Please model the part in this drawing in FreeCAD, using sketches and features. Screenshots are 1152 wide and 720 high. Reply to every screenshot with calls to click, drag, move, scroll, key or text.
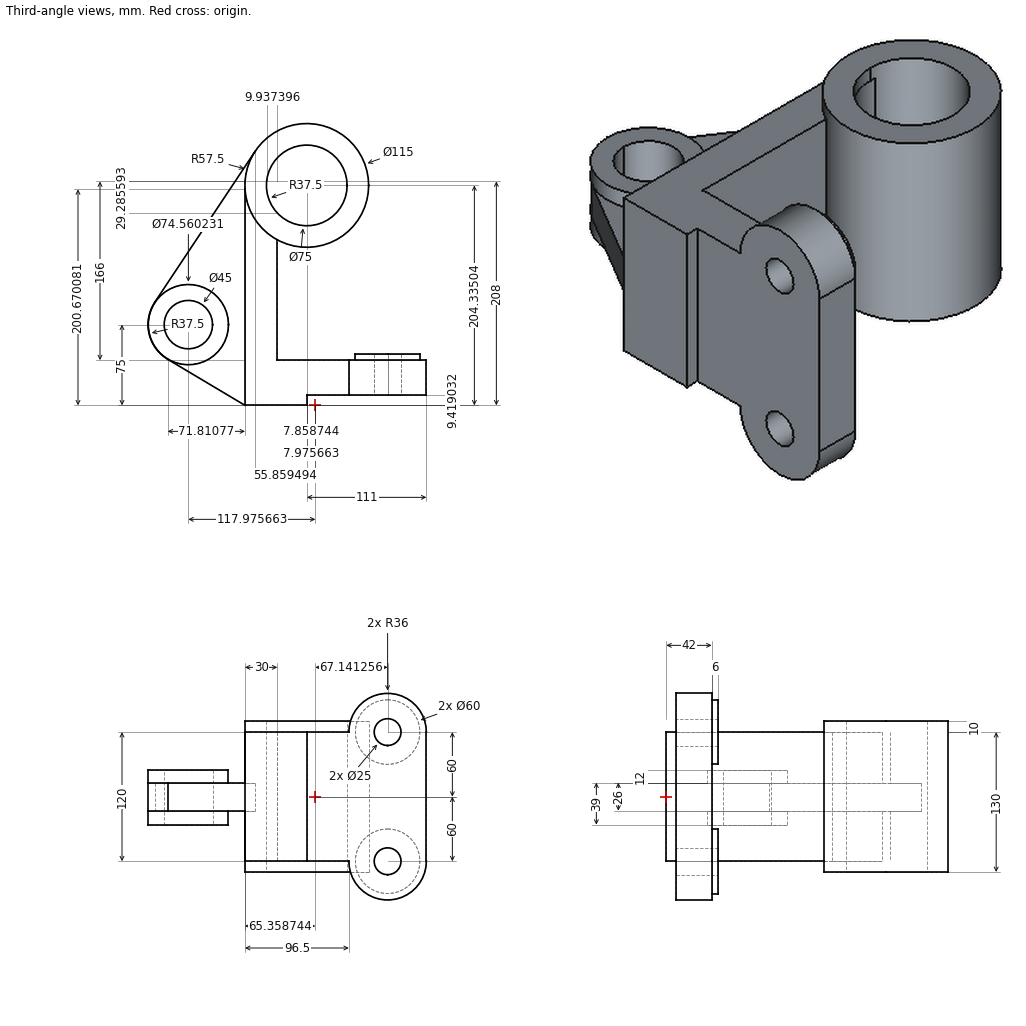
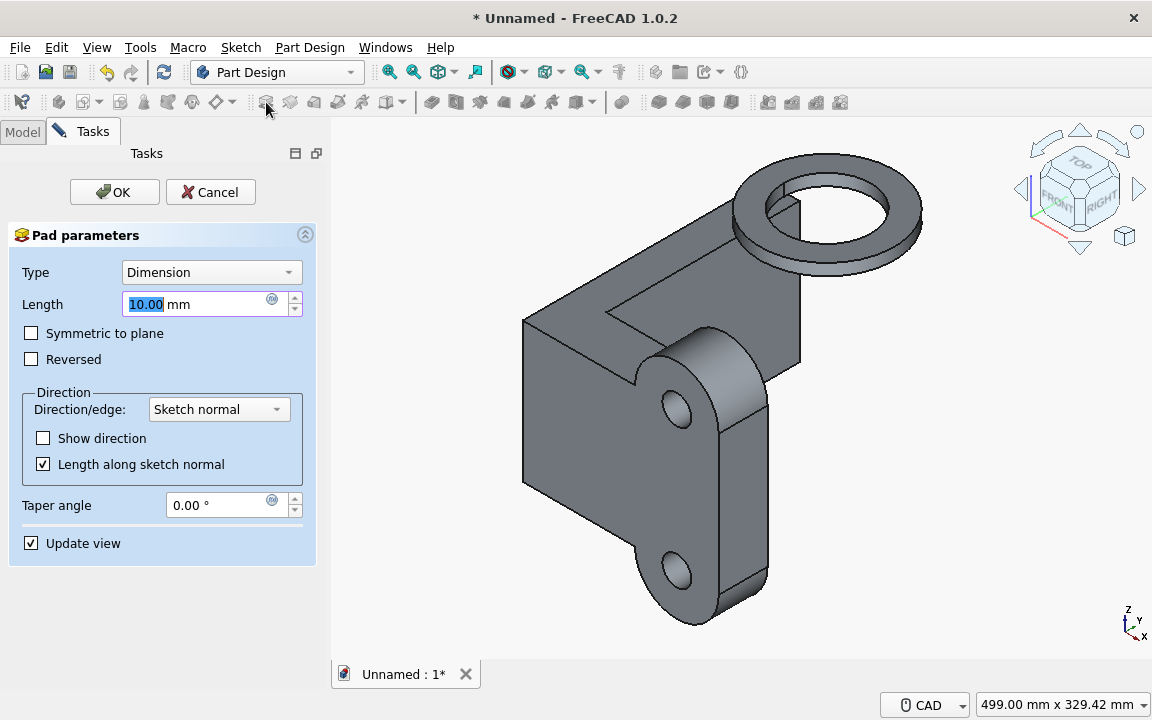
click(212, 272)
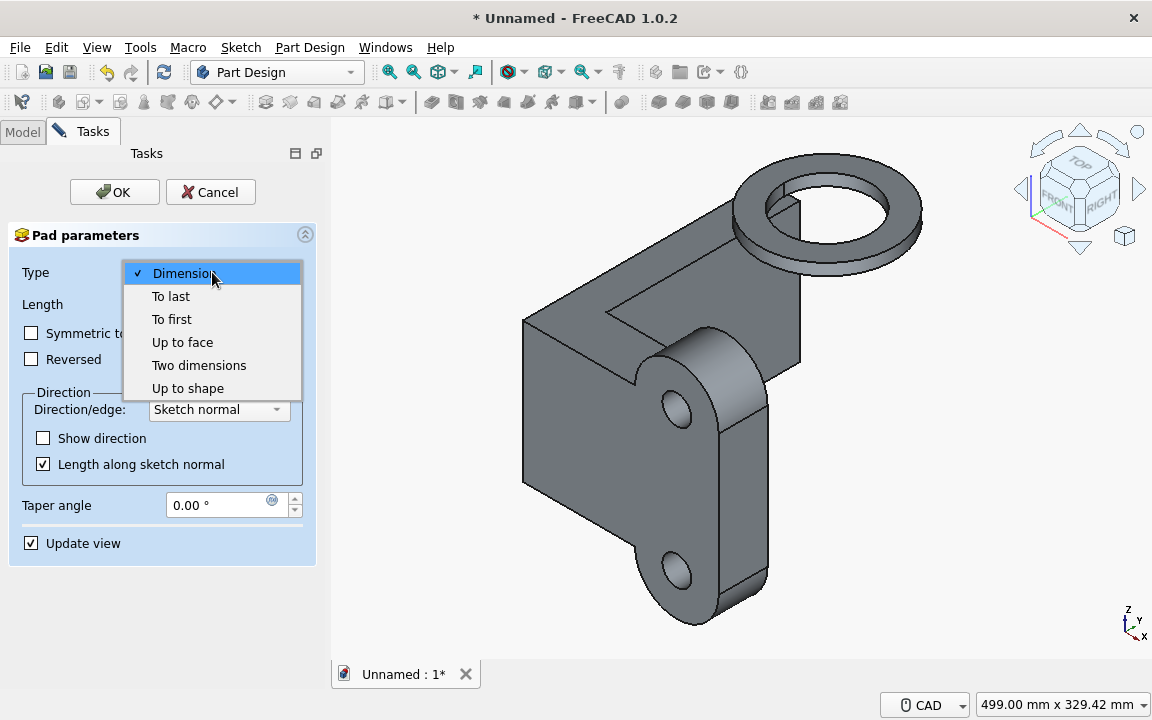
click(212, 366)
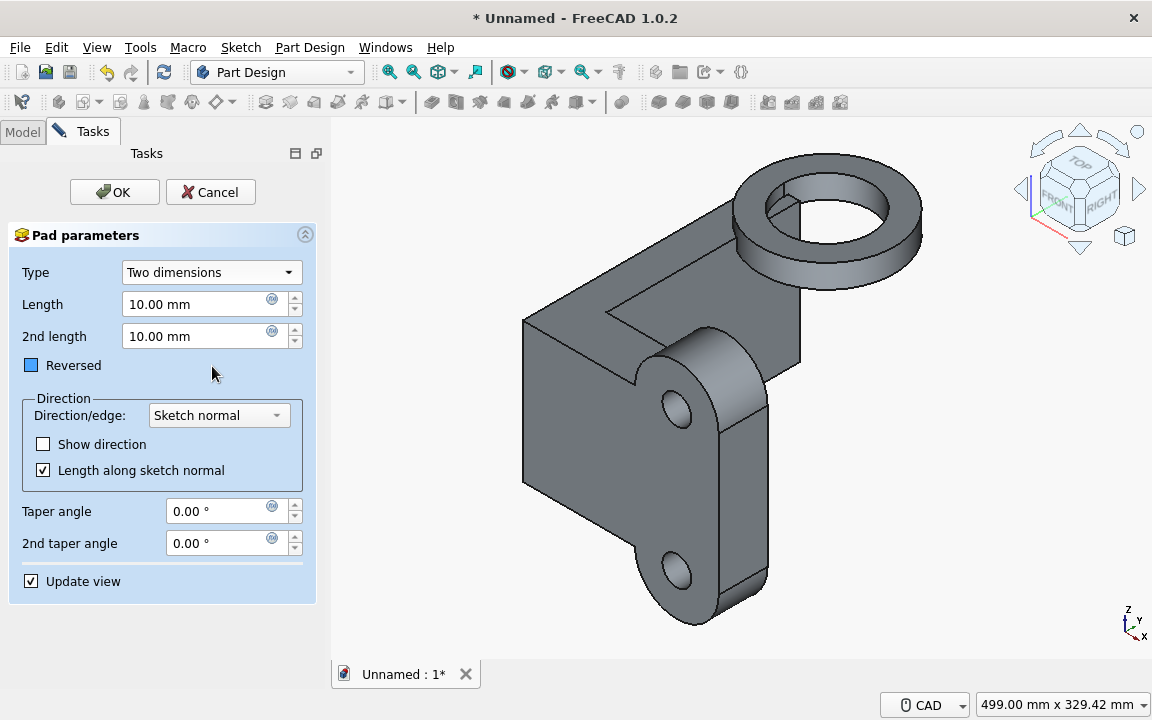
triple_click(204, 304)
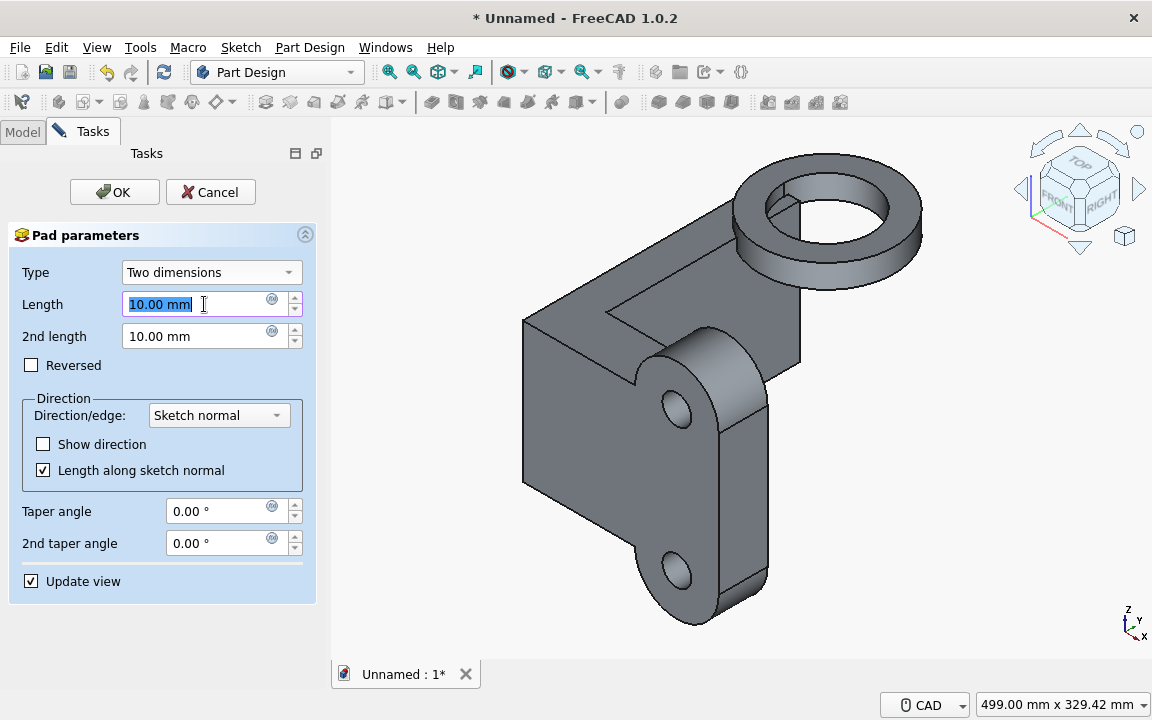
text(10)
key(Tab)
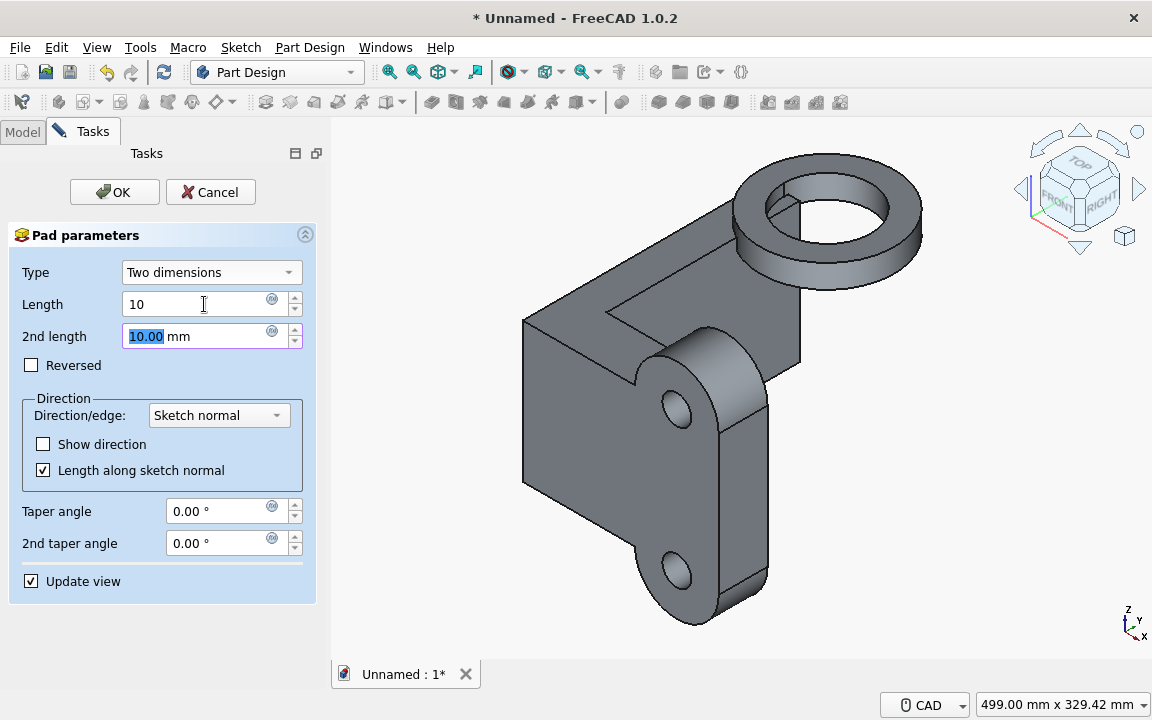
text(130)
key(Tab)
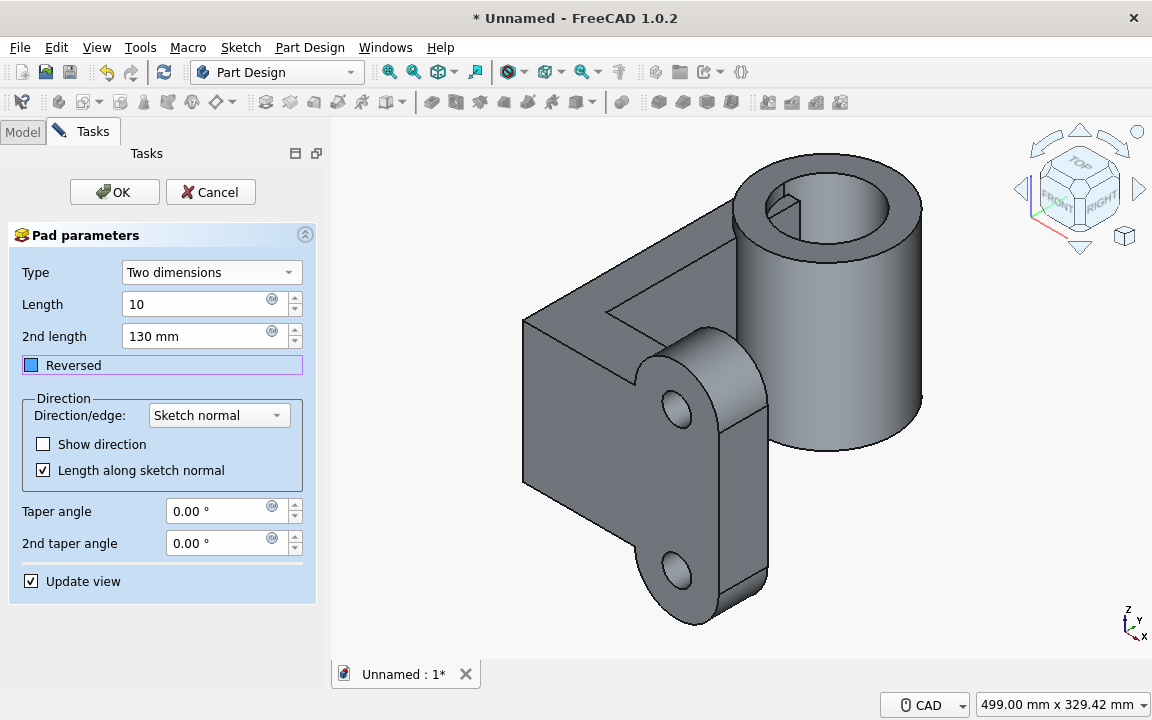
click(115, 192)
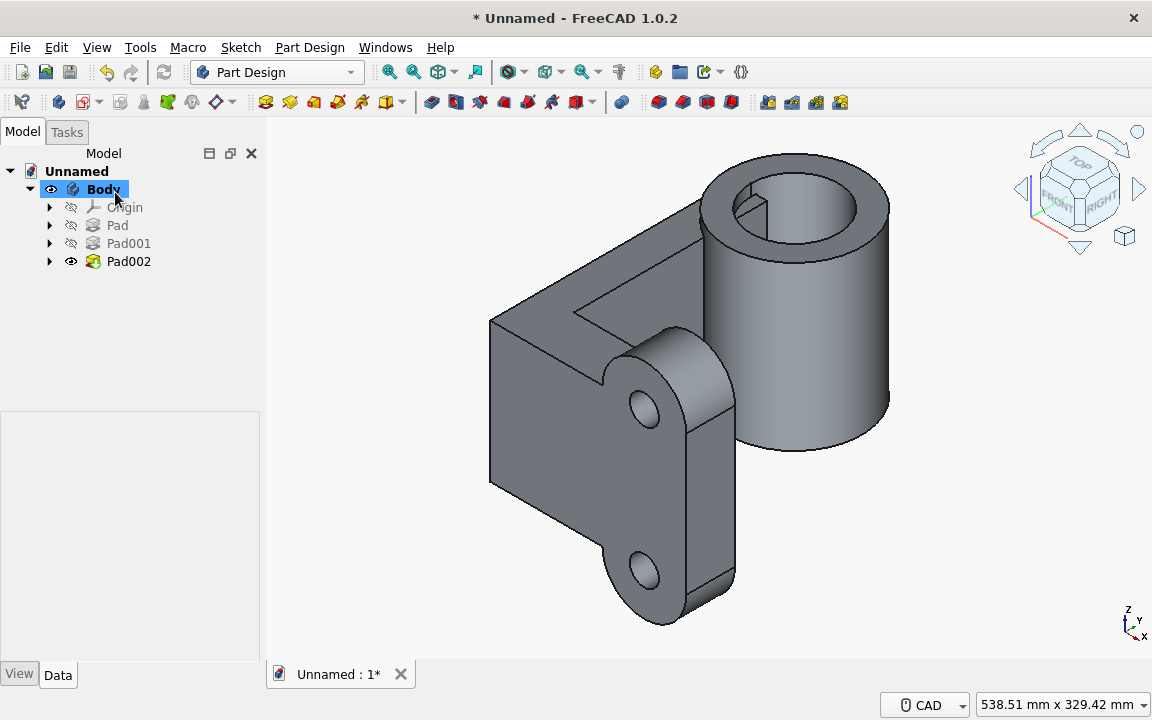
click(390, 72)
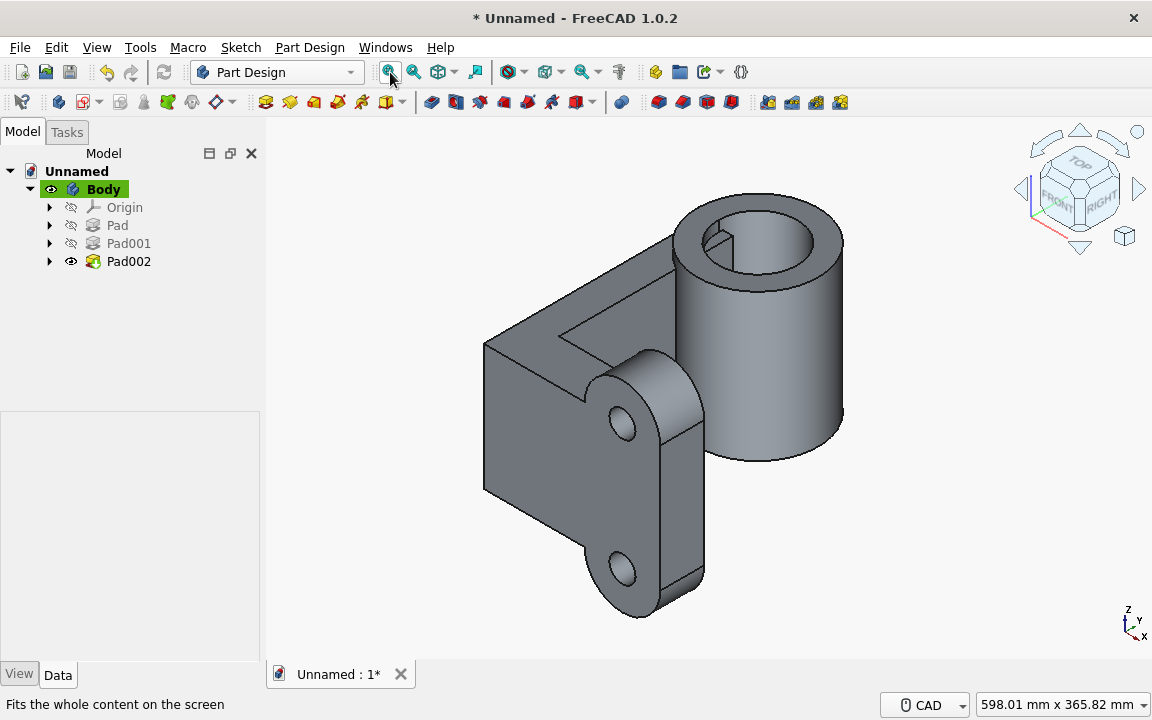
click(578, 380)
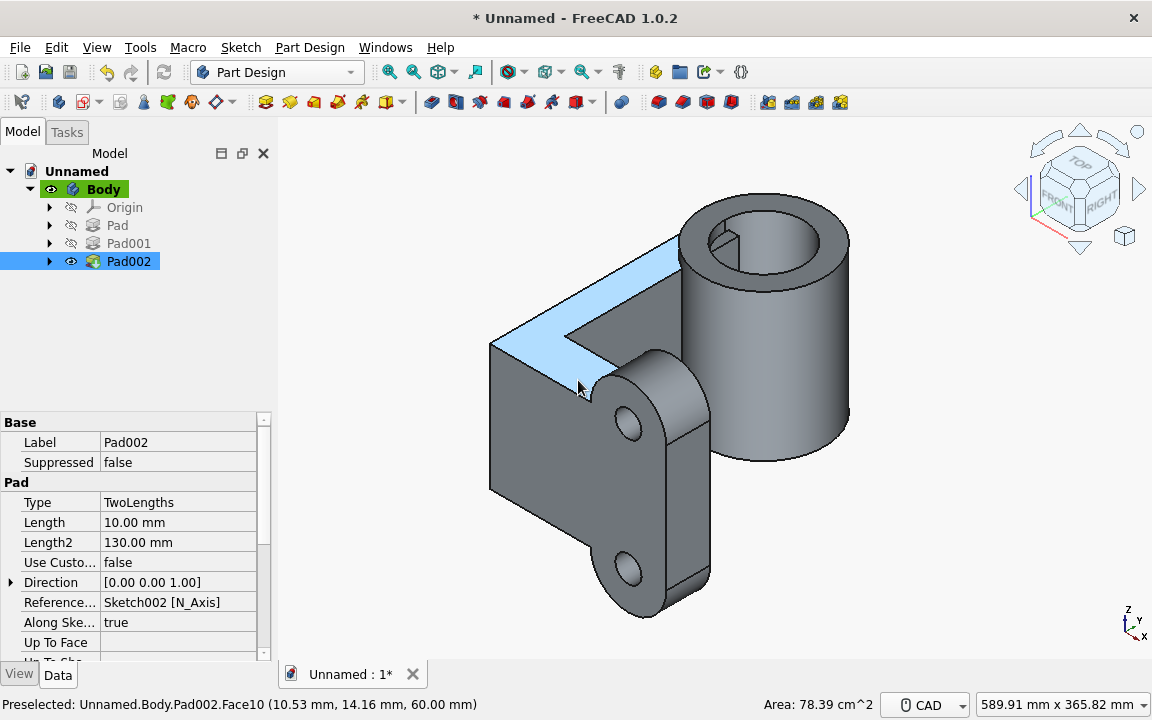
click(84, 102)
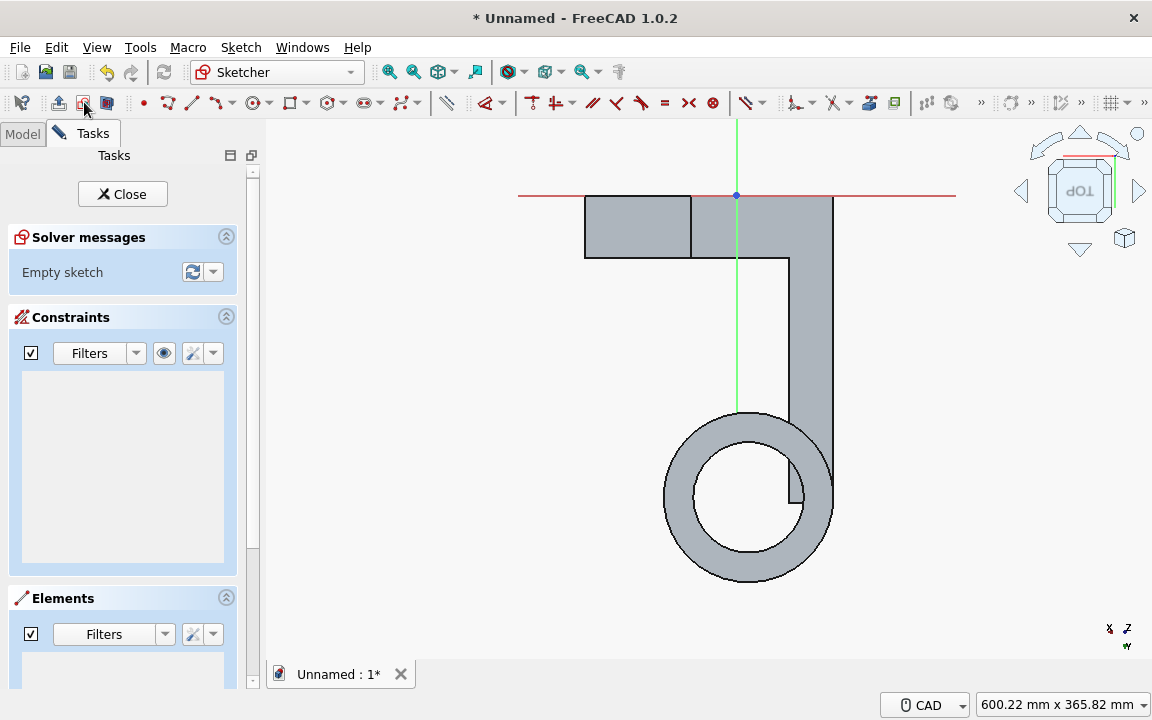
scroll(821, 496, up, 10)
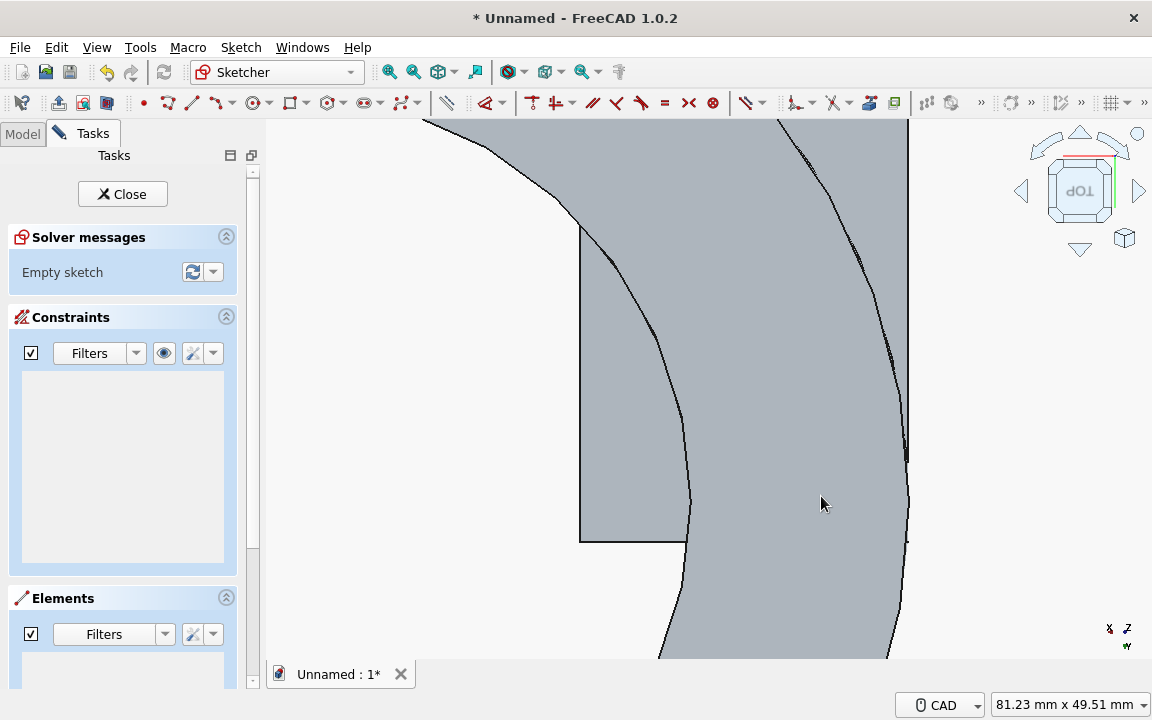
click(168, 104)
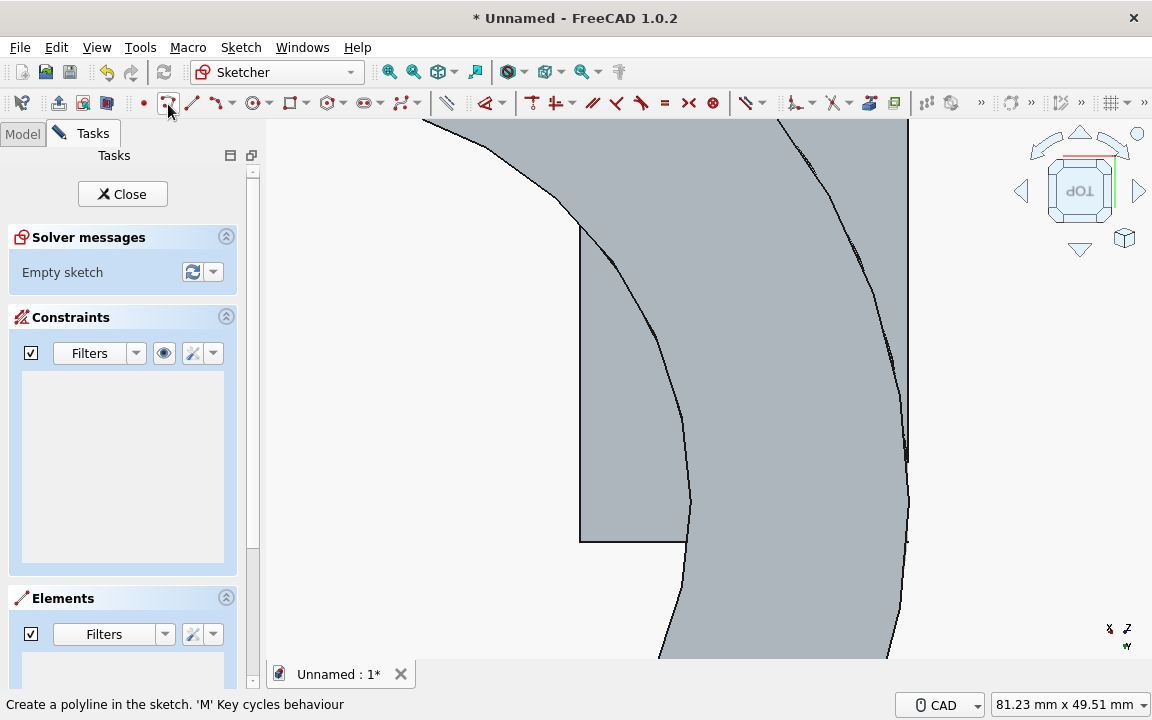
click(580, 223)
click(580, 542)
click(689, 542)
right_click(689, 542)